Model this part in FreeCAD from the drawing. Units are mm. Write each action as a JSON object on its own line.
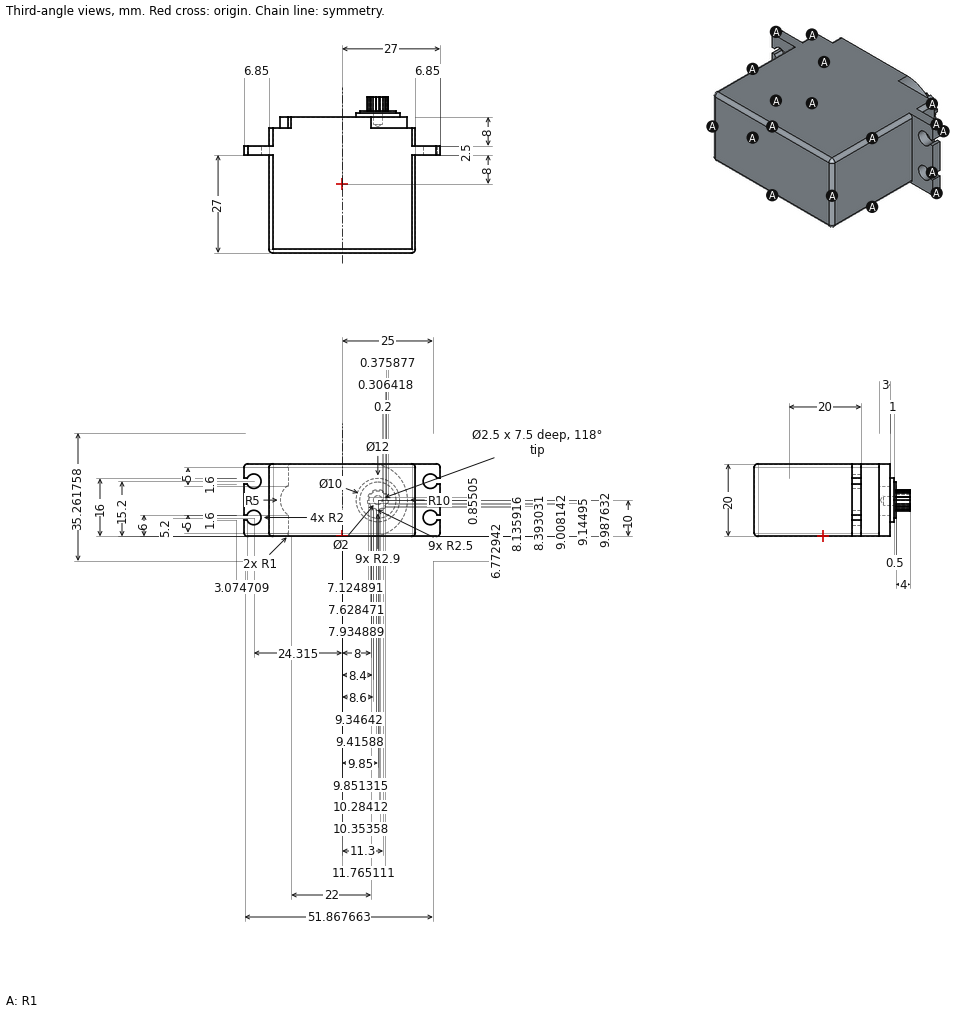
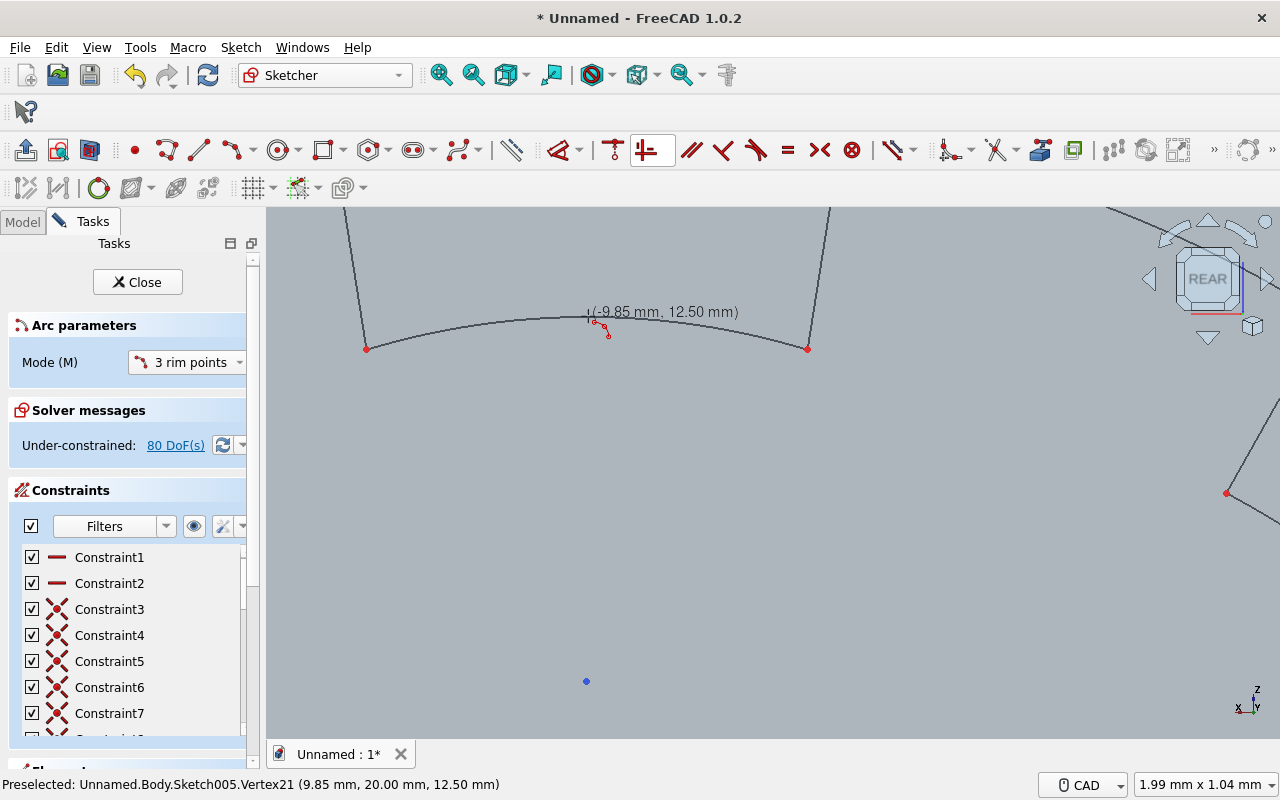
{"action": "scroll", "coordinate": [618, 319], "scroll_direction": "down", "scroll_amount": 15}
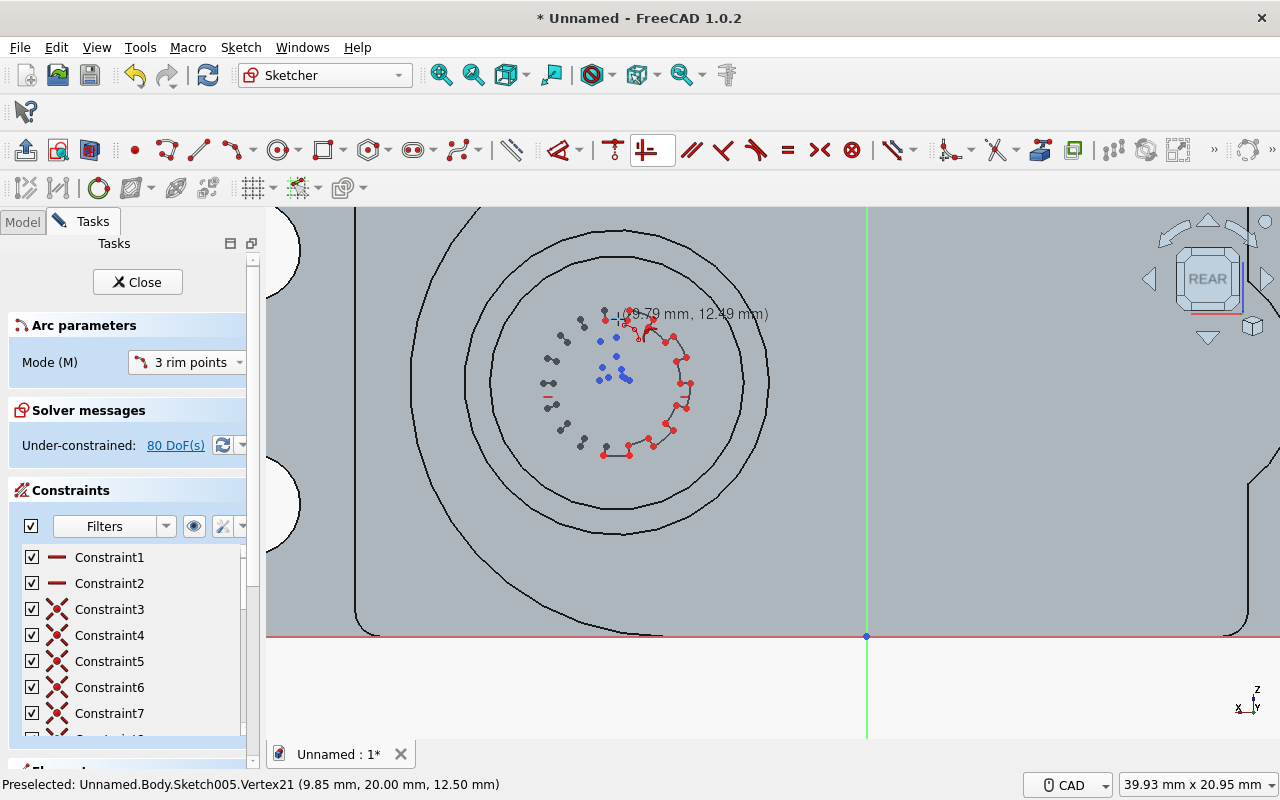
{"action": "scroll", "coordinate": [604, 310], "scroll_direction": "up", "scroll_amount": 6}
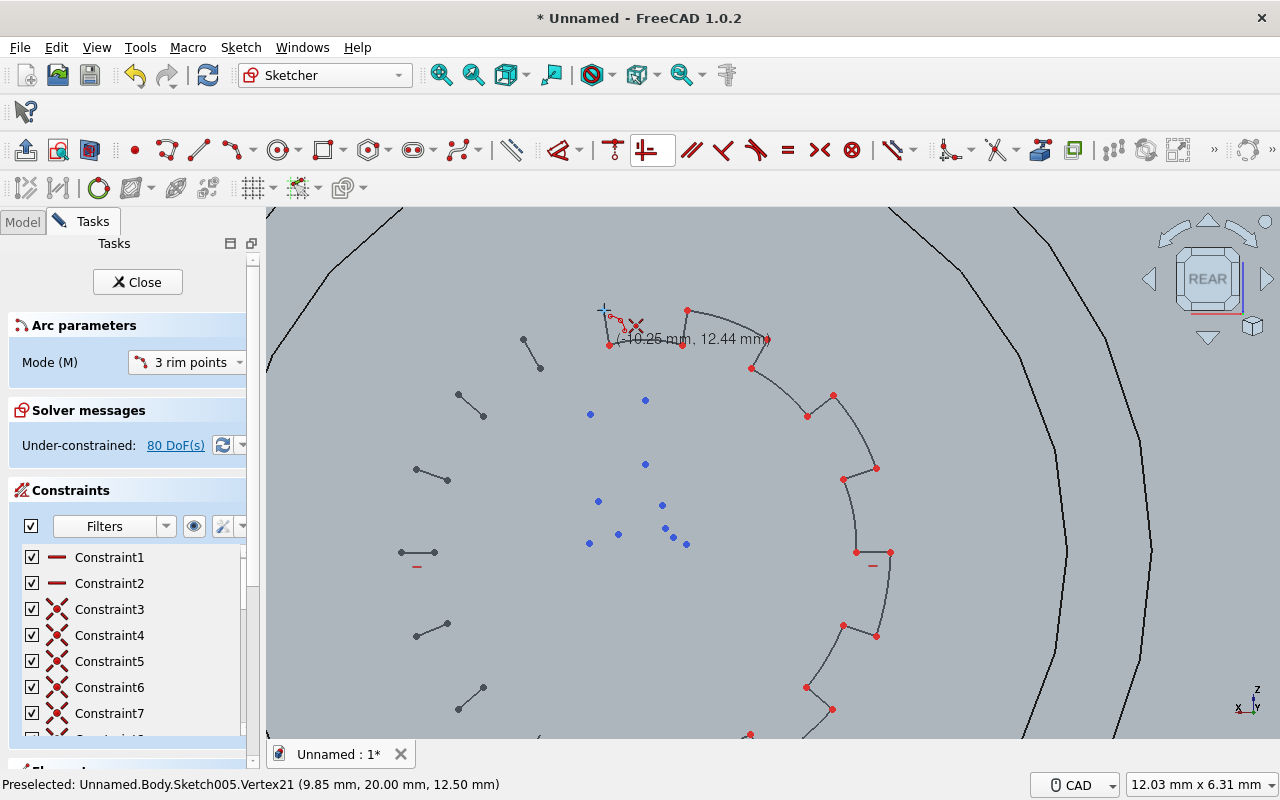
{"action": "left_click", "coordinate": [604, 311]}
{"action": "left_click", "coordinate": [524, 340]}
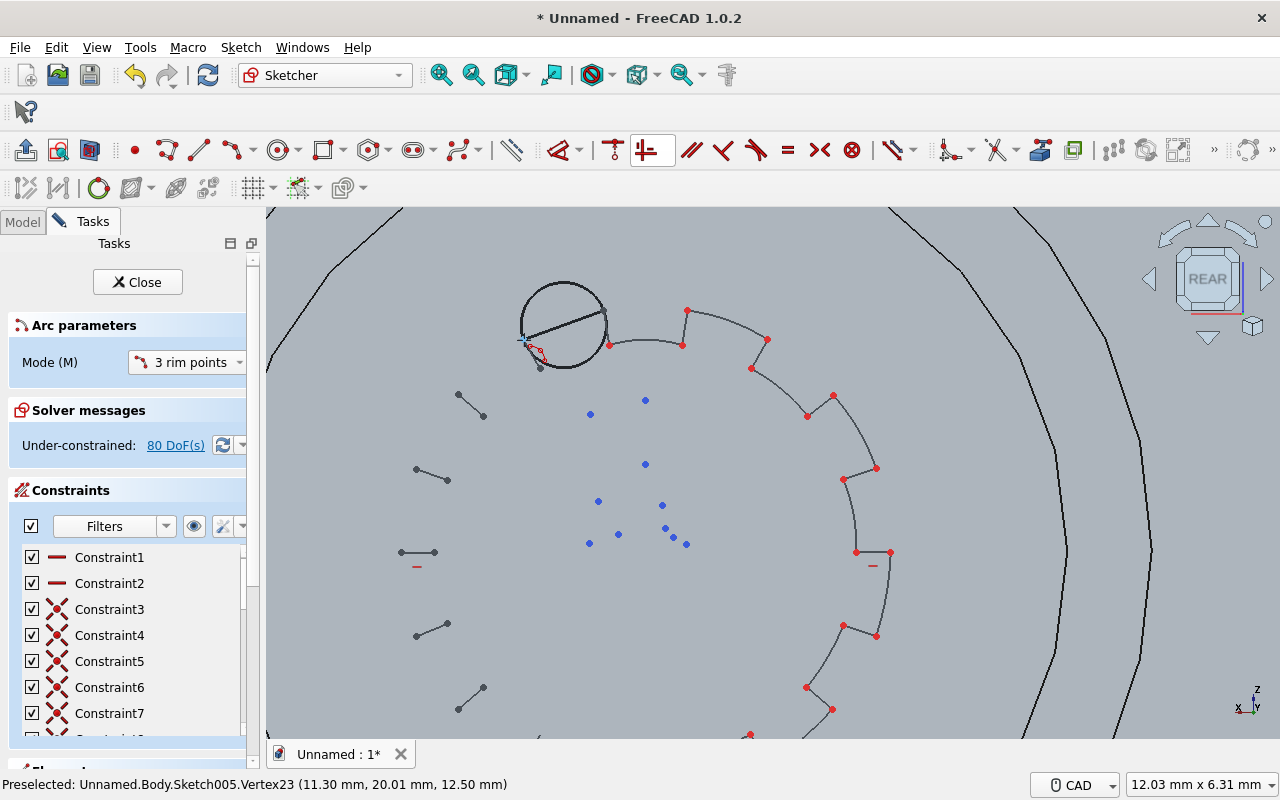
{"action": "scroll", "coordinate": [562, 321], "scroll_direction": "up", "scroll_amount": 8}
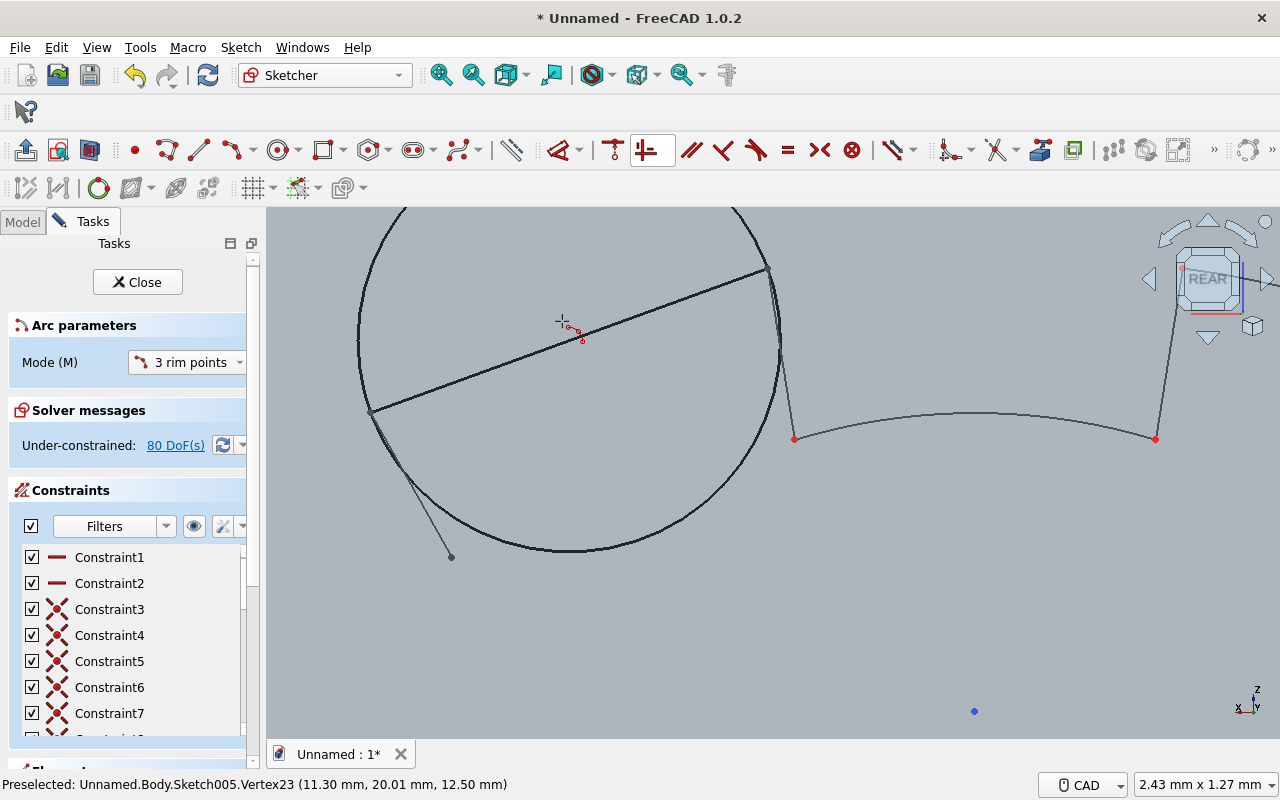
{"action": "left_click", "coordinate": [562, 319]}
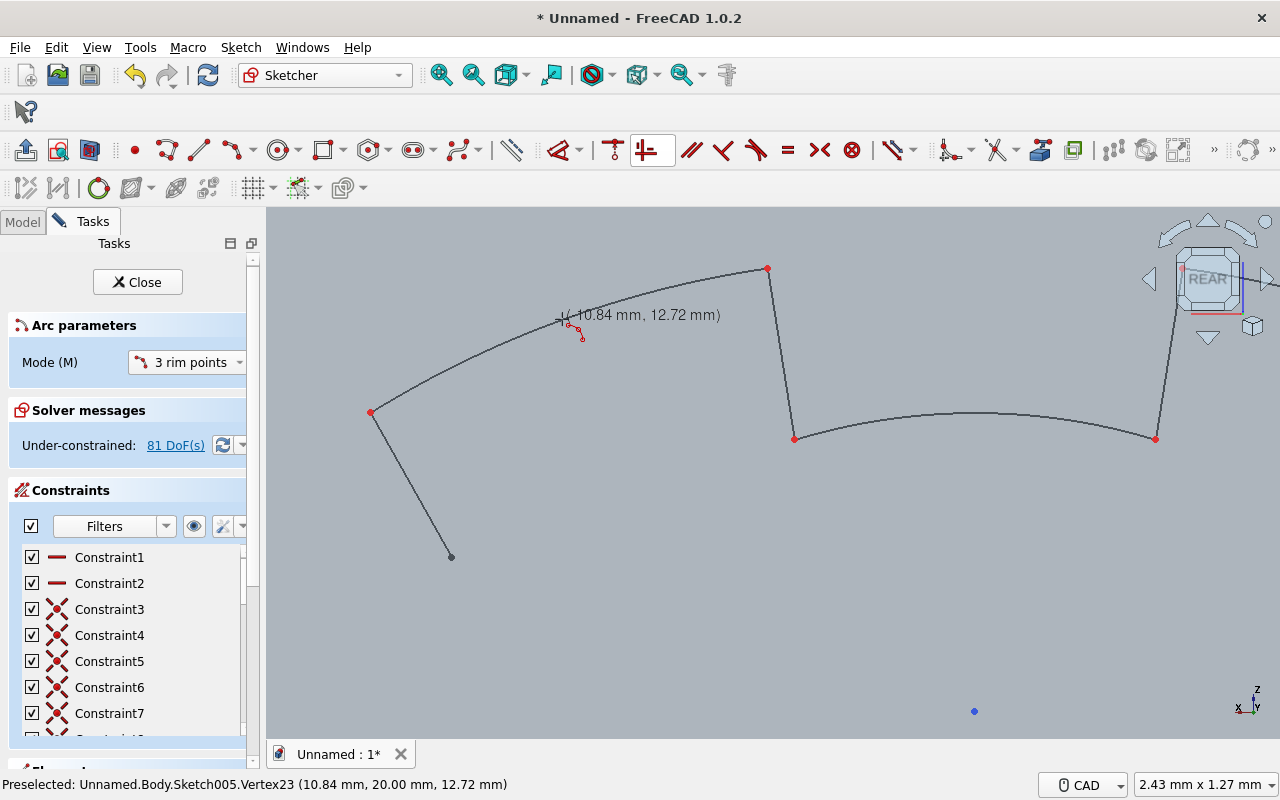
{"action": "scroll", "coordinate": [593, 313], "scroll_direction": "down", "scroll_amount": 14}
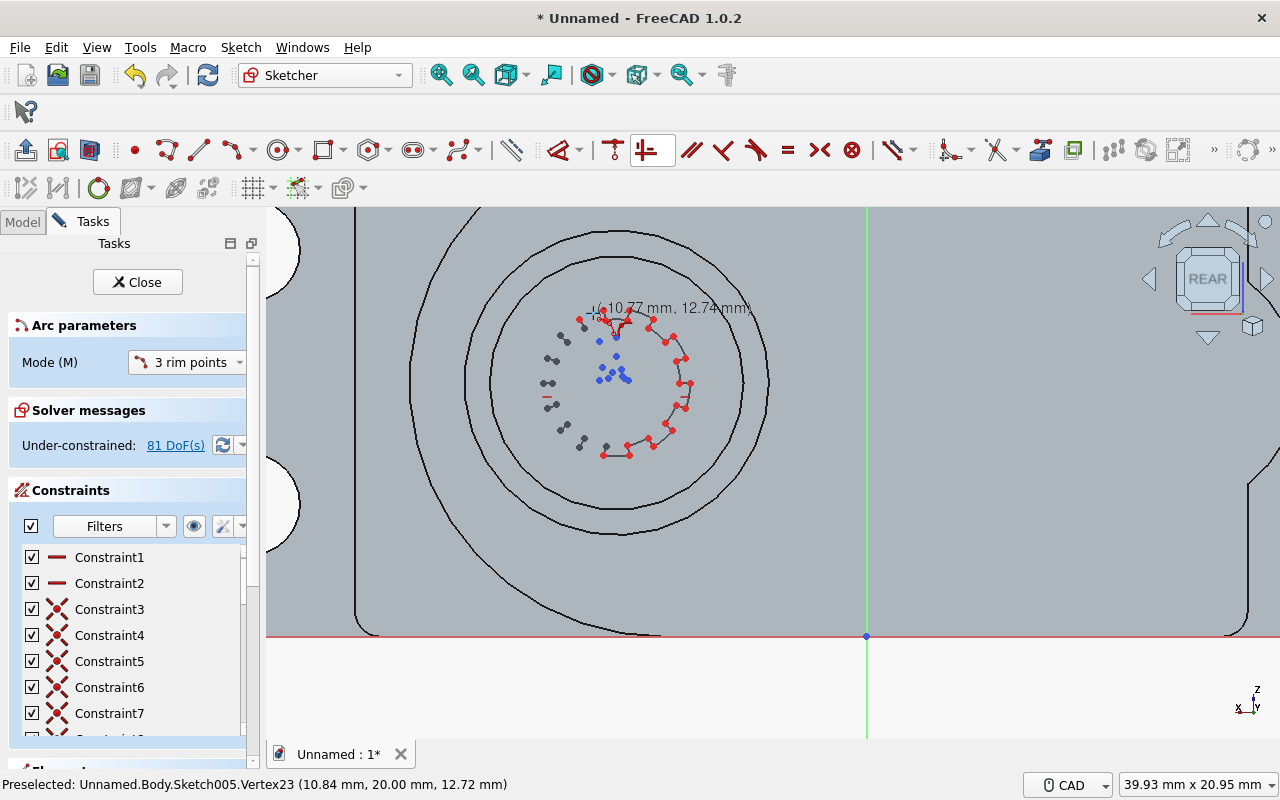
{"action": "scroll", "coordinate": [585, 328], "scroll_direction": "up", "scroll_amount": 6}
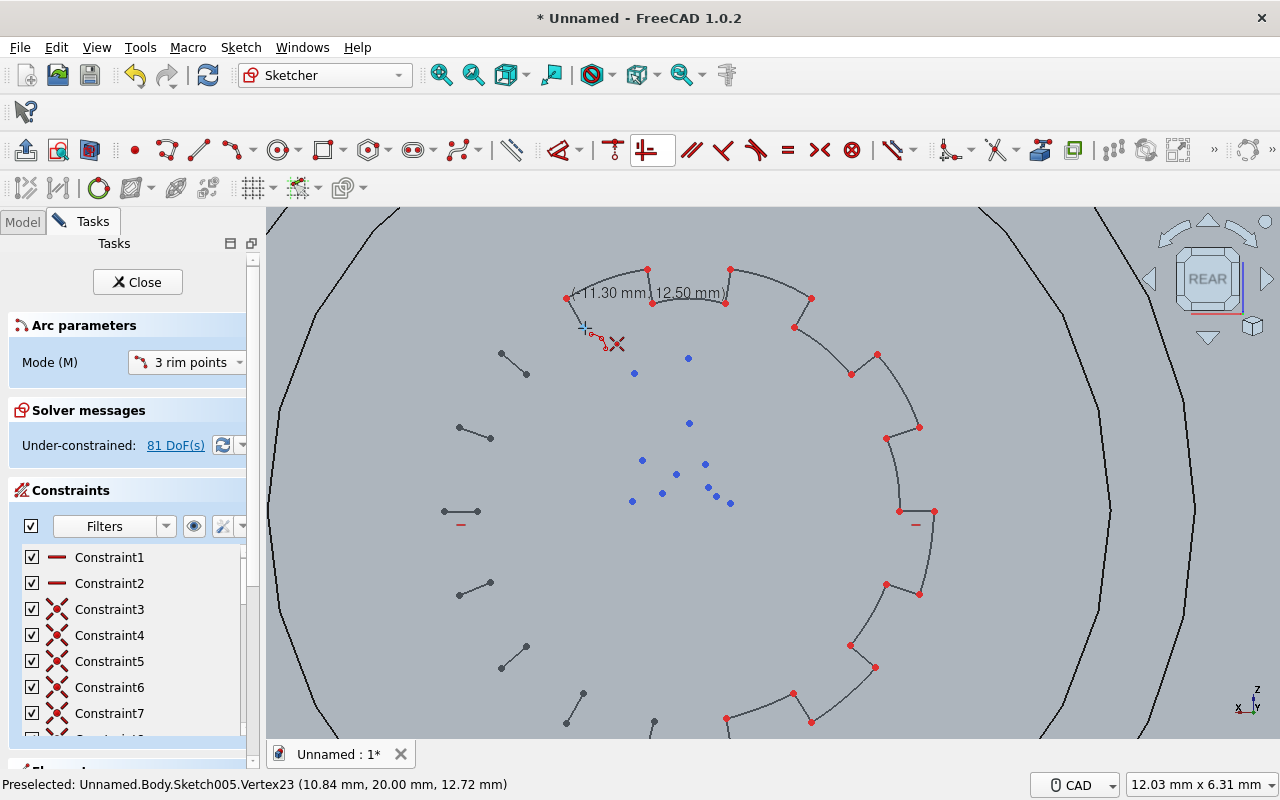
{"action": "left_click", "coordinate": [583, 328]}
{"action": "left_click", "coordinate": [527, 375]}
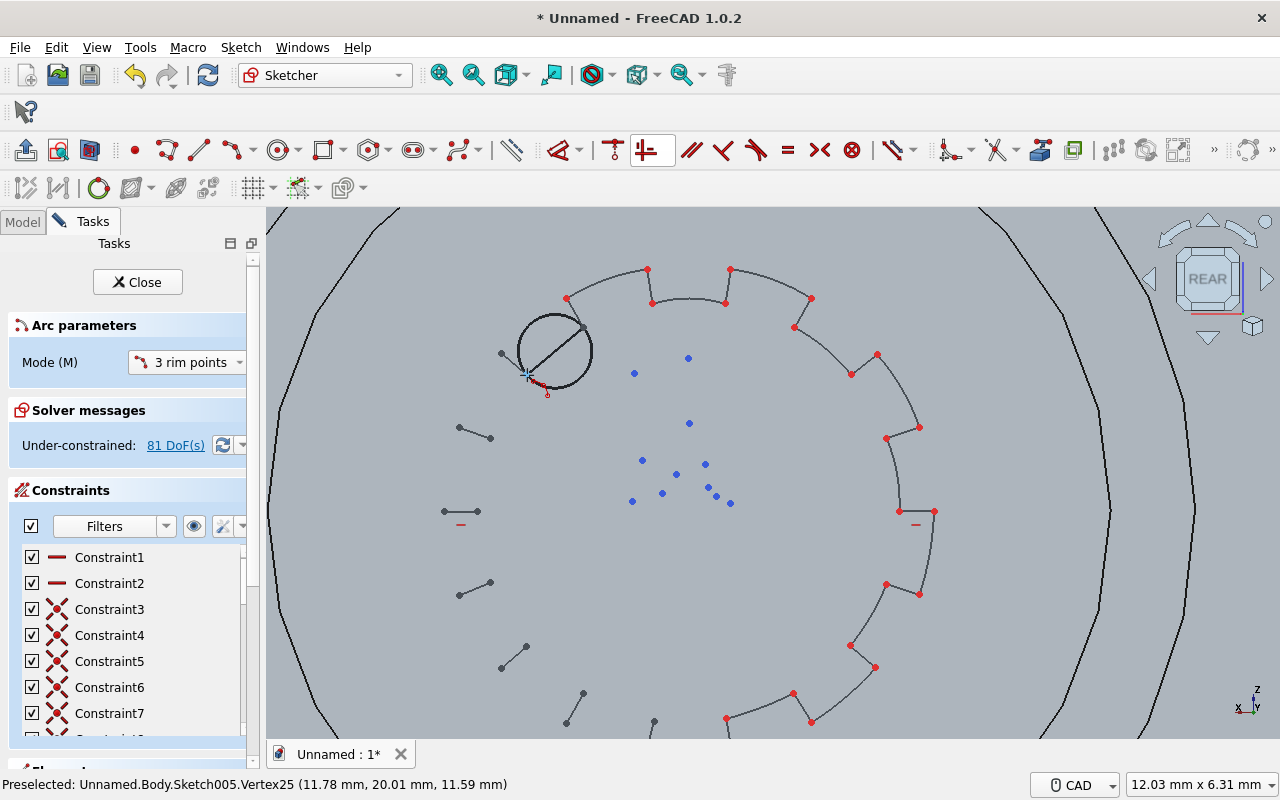
{"action": "scroll", "coordinate": [554, 348], "scroll_direction": "up", "scroll_amount": 9}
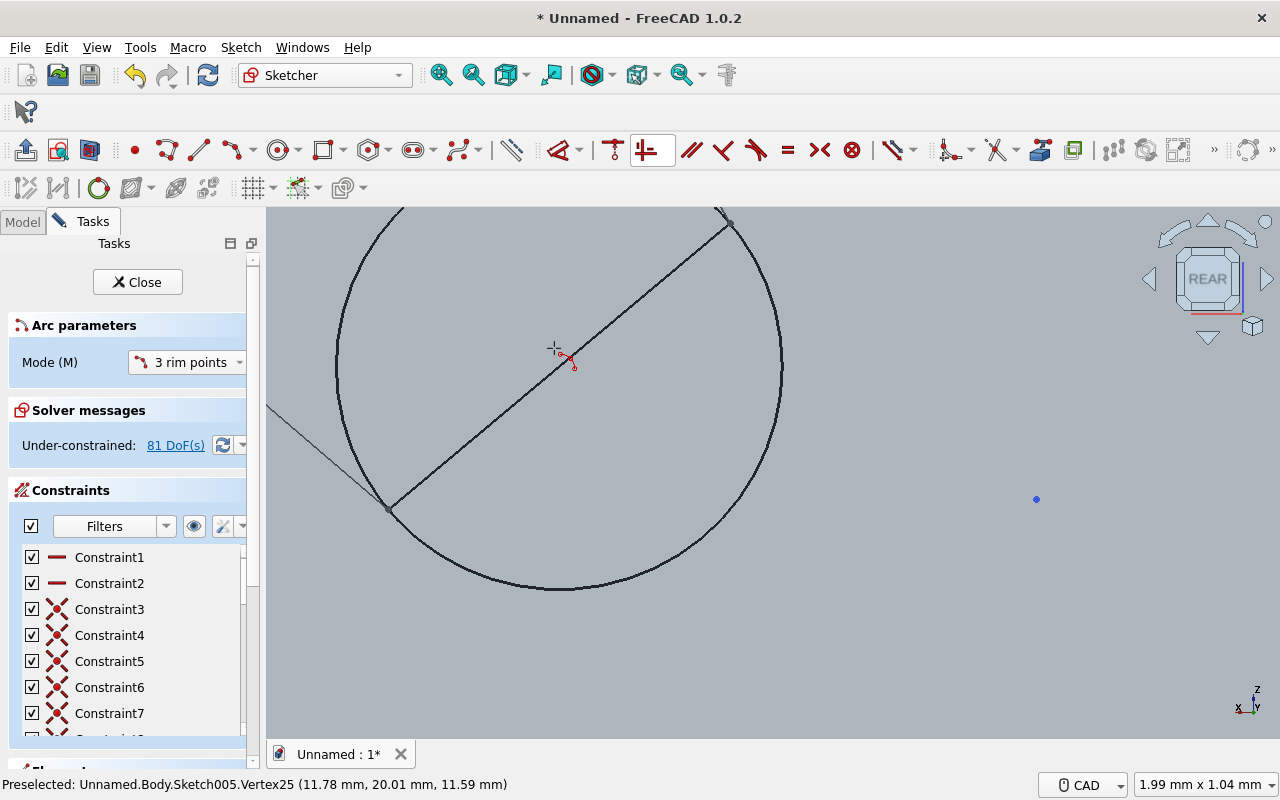
{"action": "left_click", "coordinate": [551, 345]}